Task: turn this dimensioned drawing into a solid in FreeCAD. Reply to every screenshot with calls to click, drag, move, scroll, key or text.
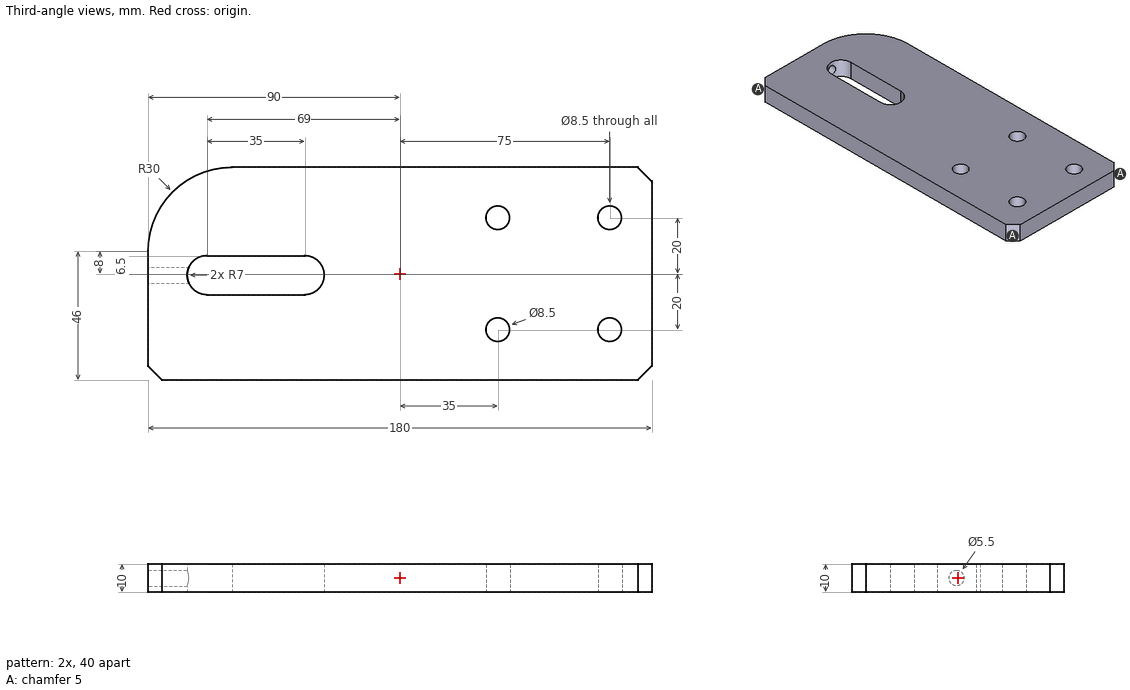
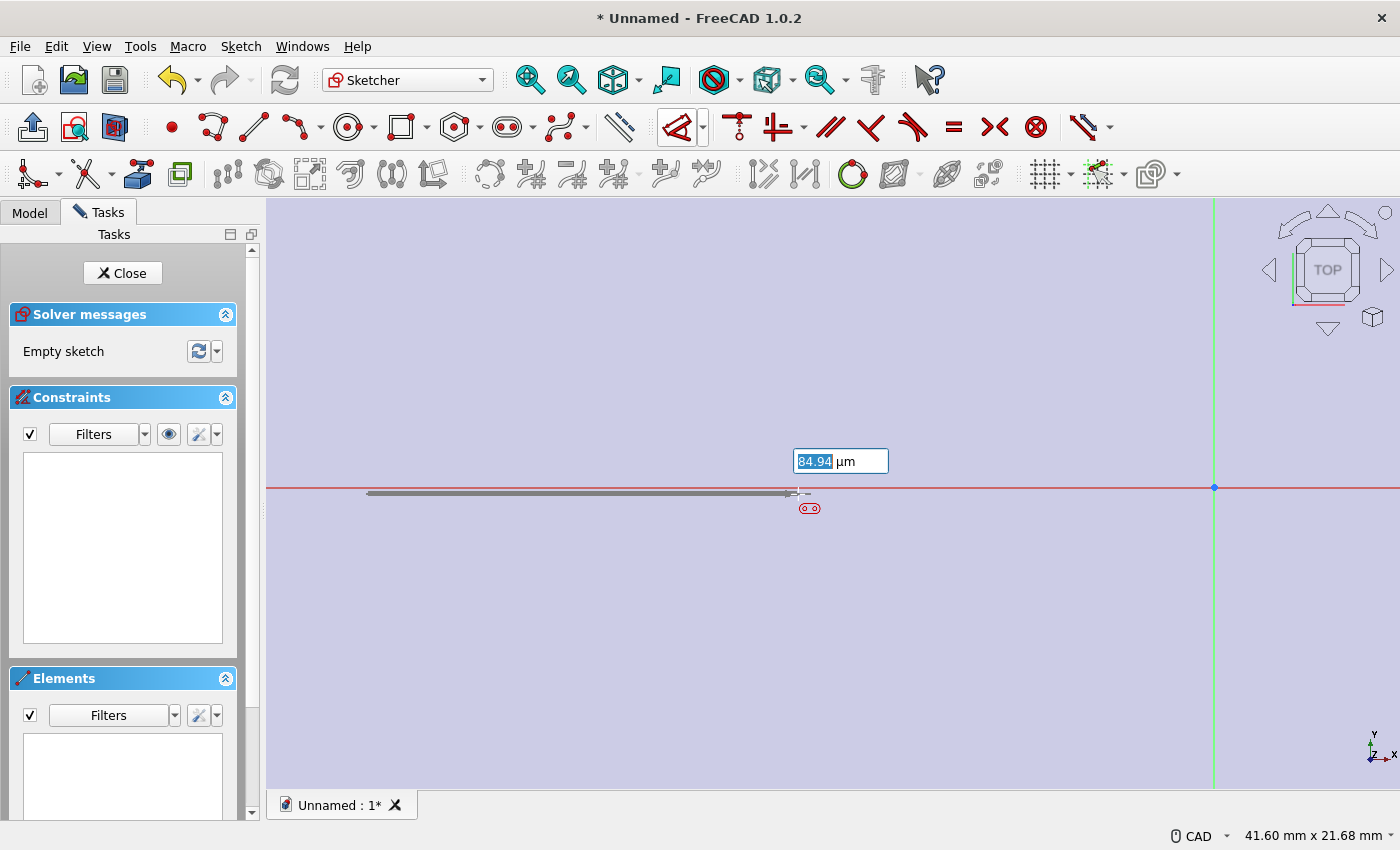
click(654, 436)
key(Escape)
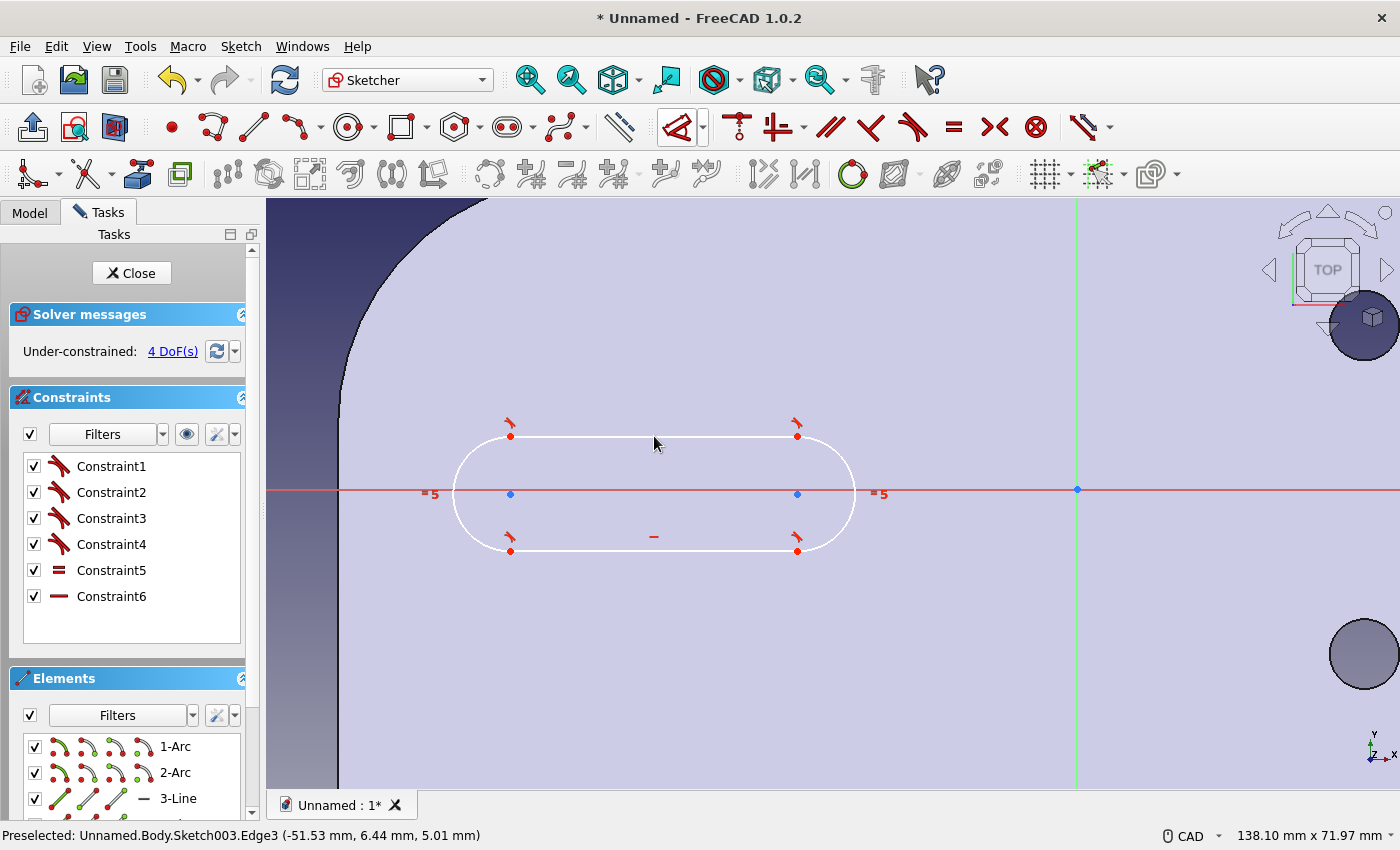
click(464, 461)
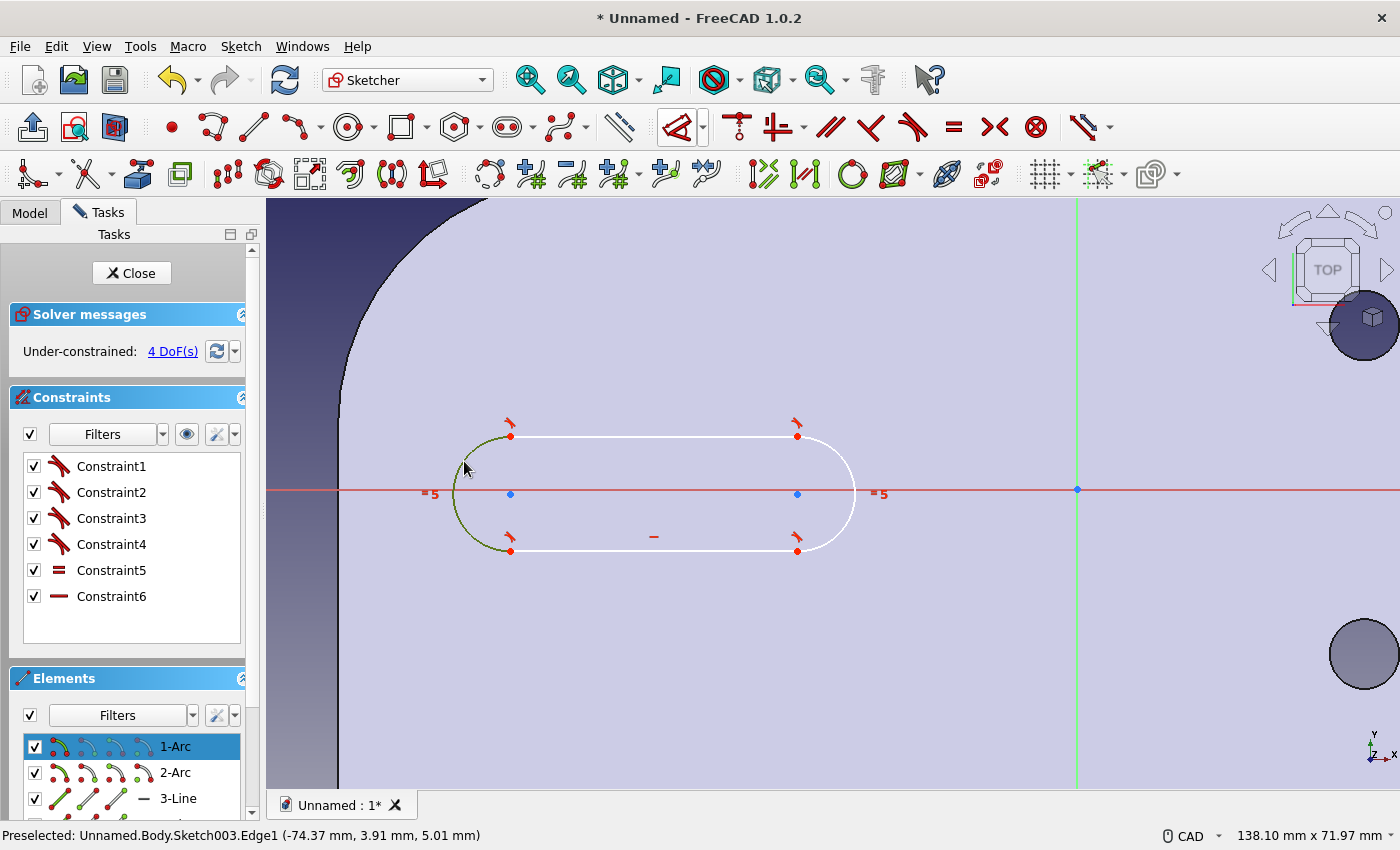
key(k)
key(r)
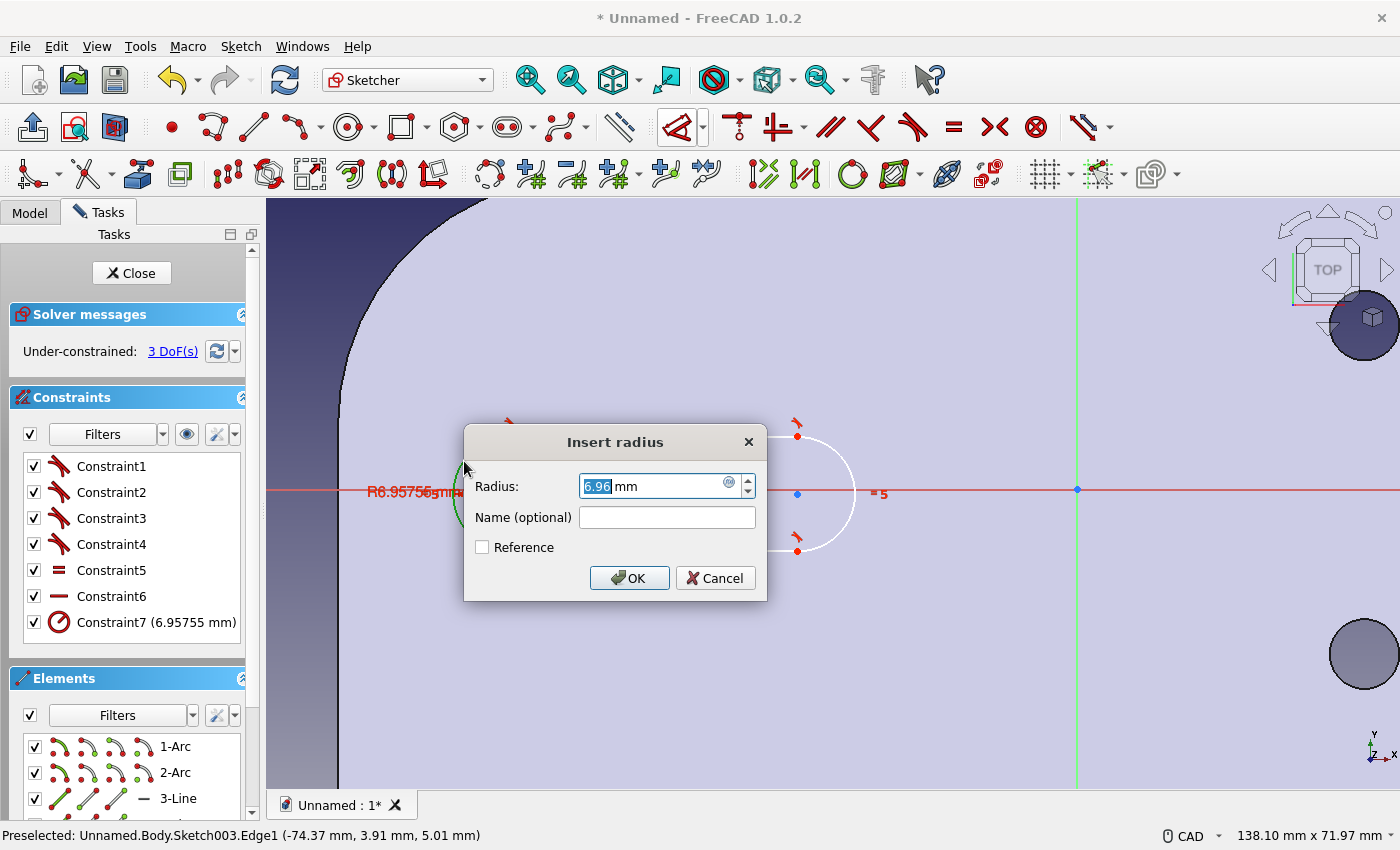
text(7)
key(Return)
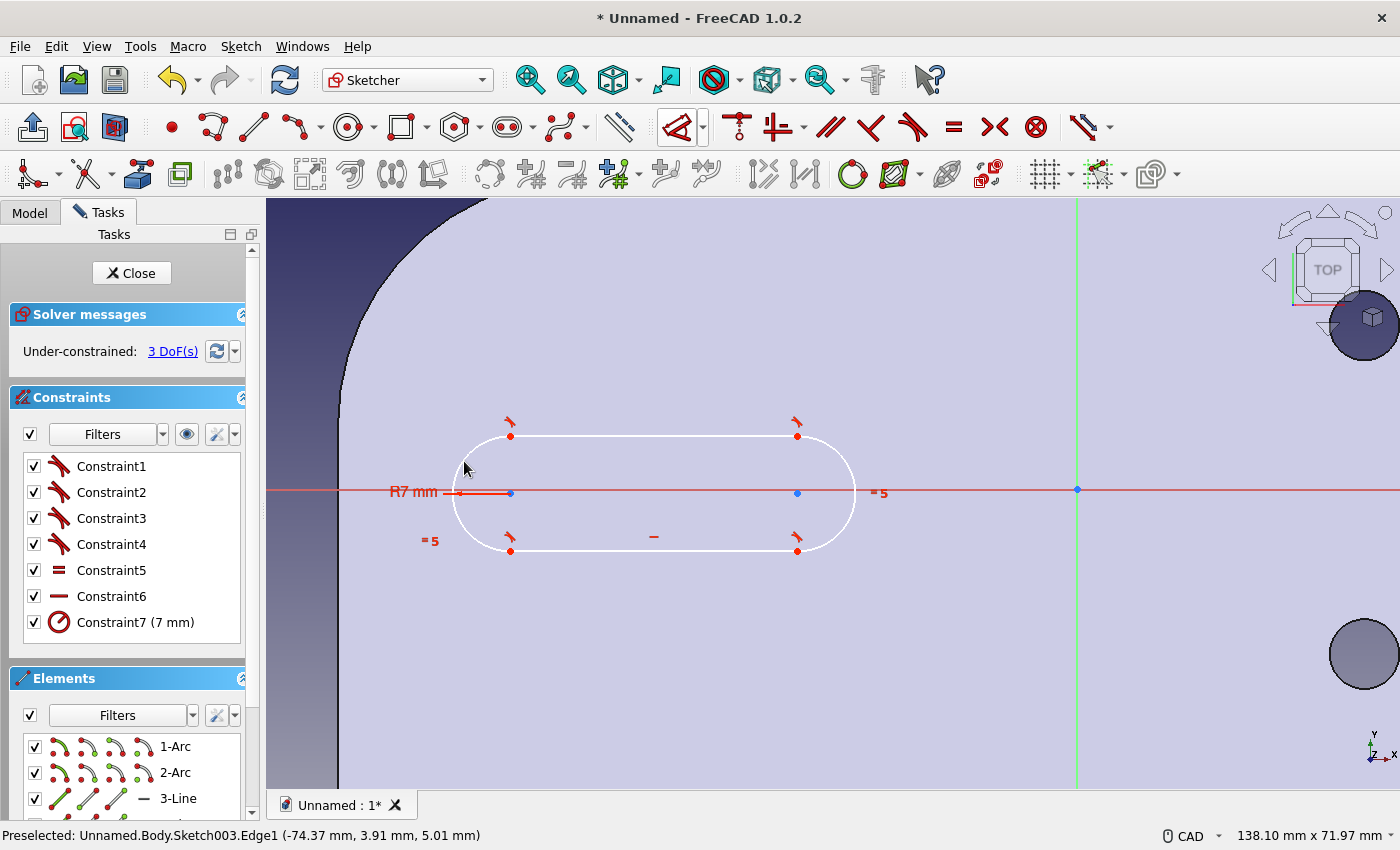
click(597, 436)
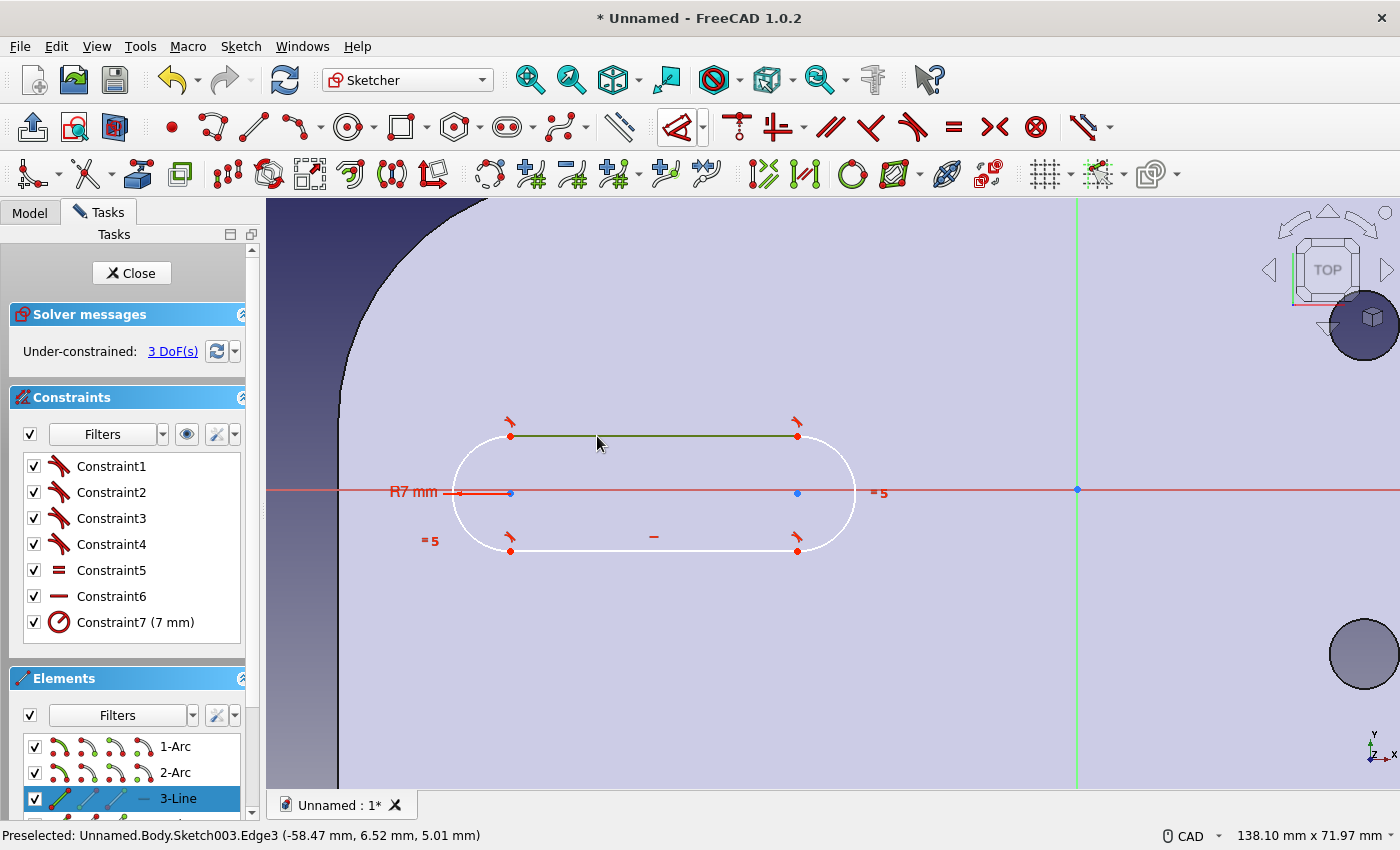
key(l)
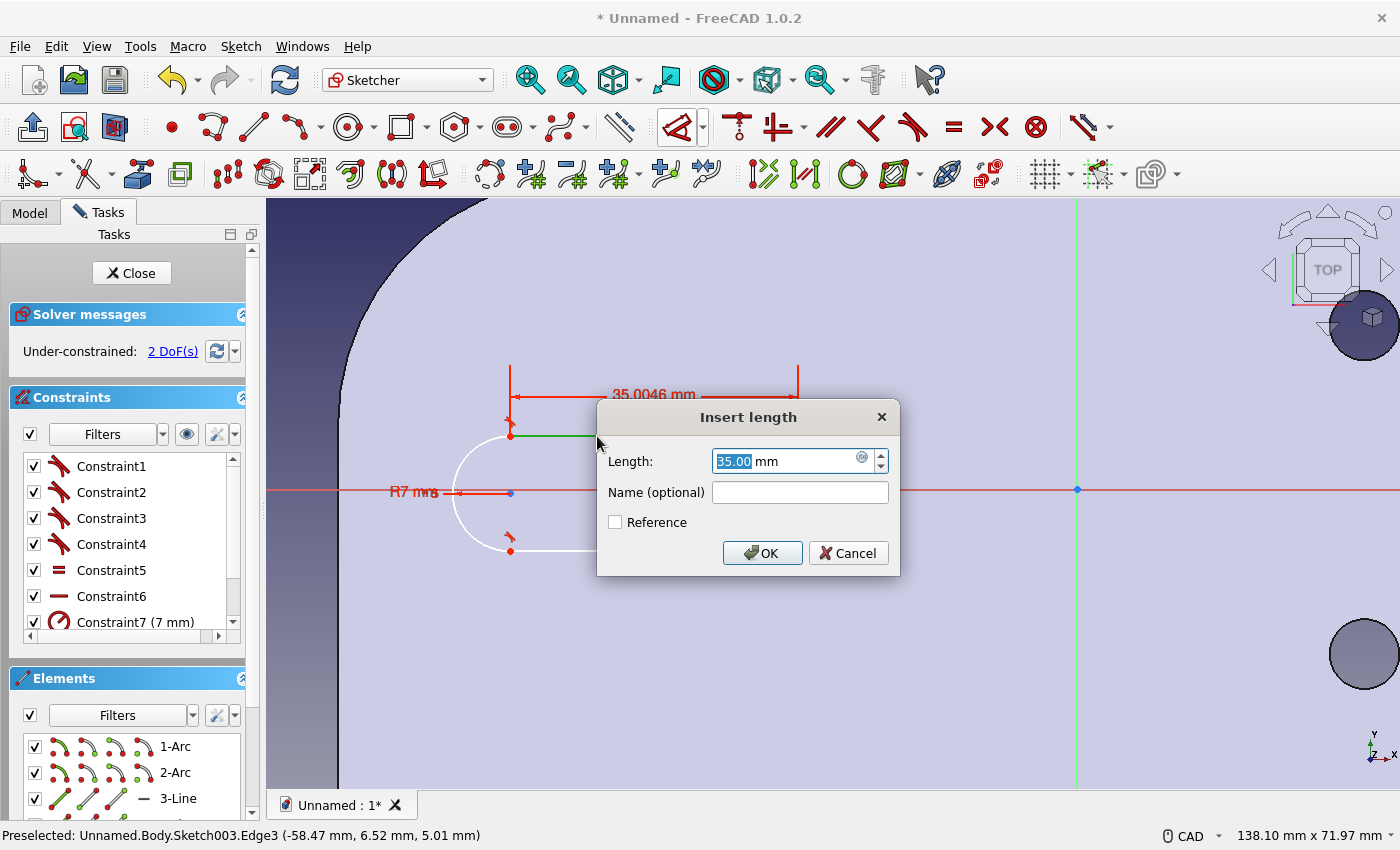
text(35)
key(Return)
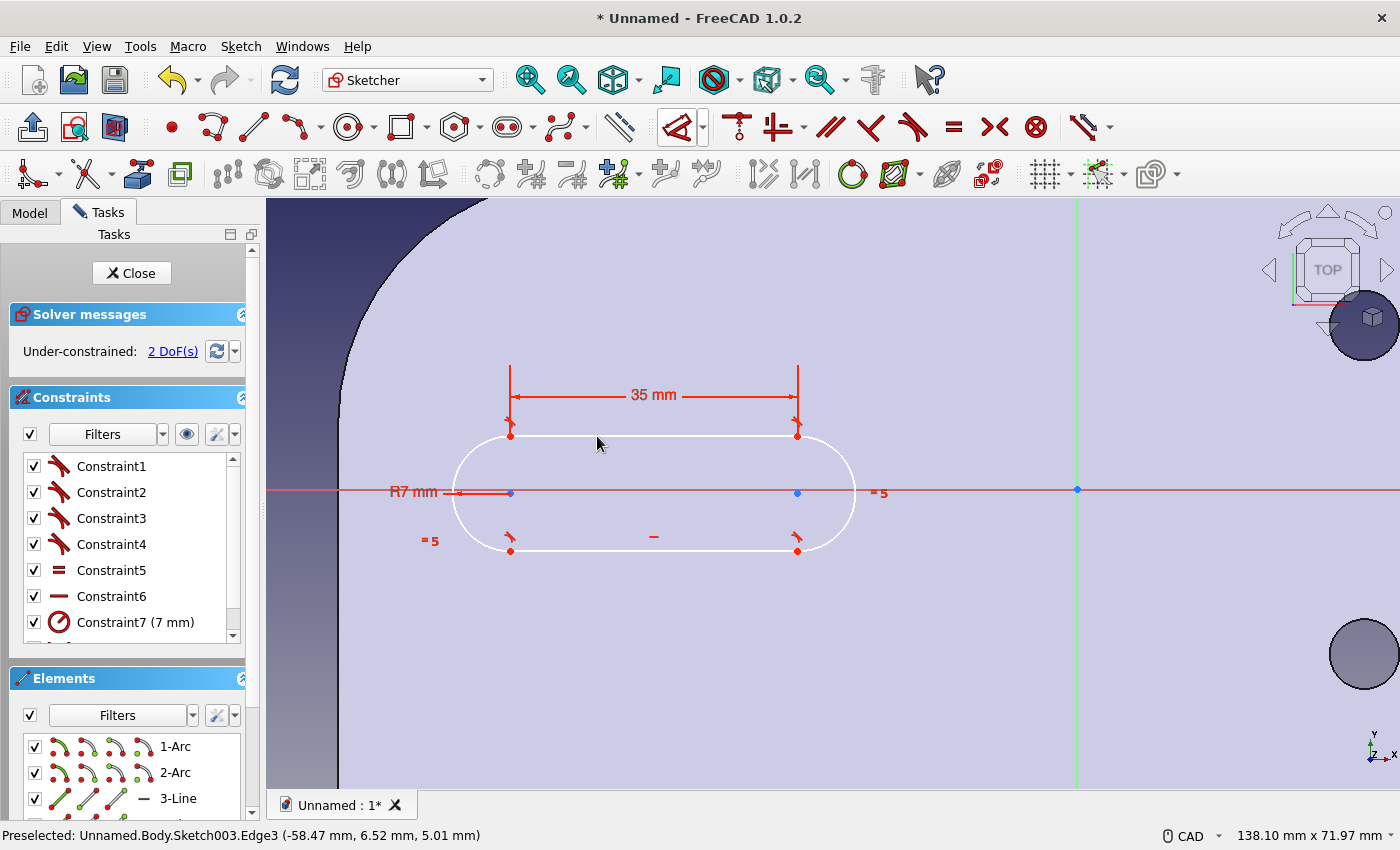
click(510, 436)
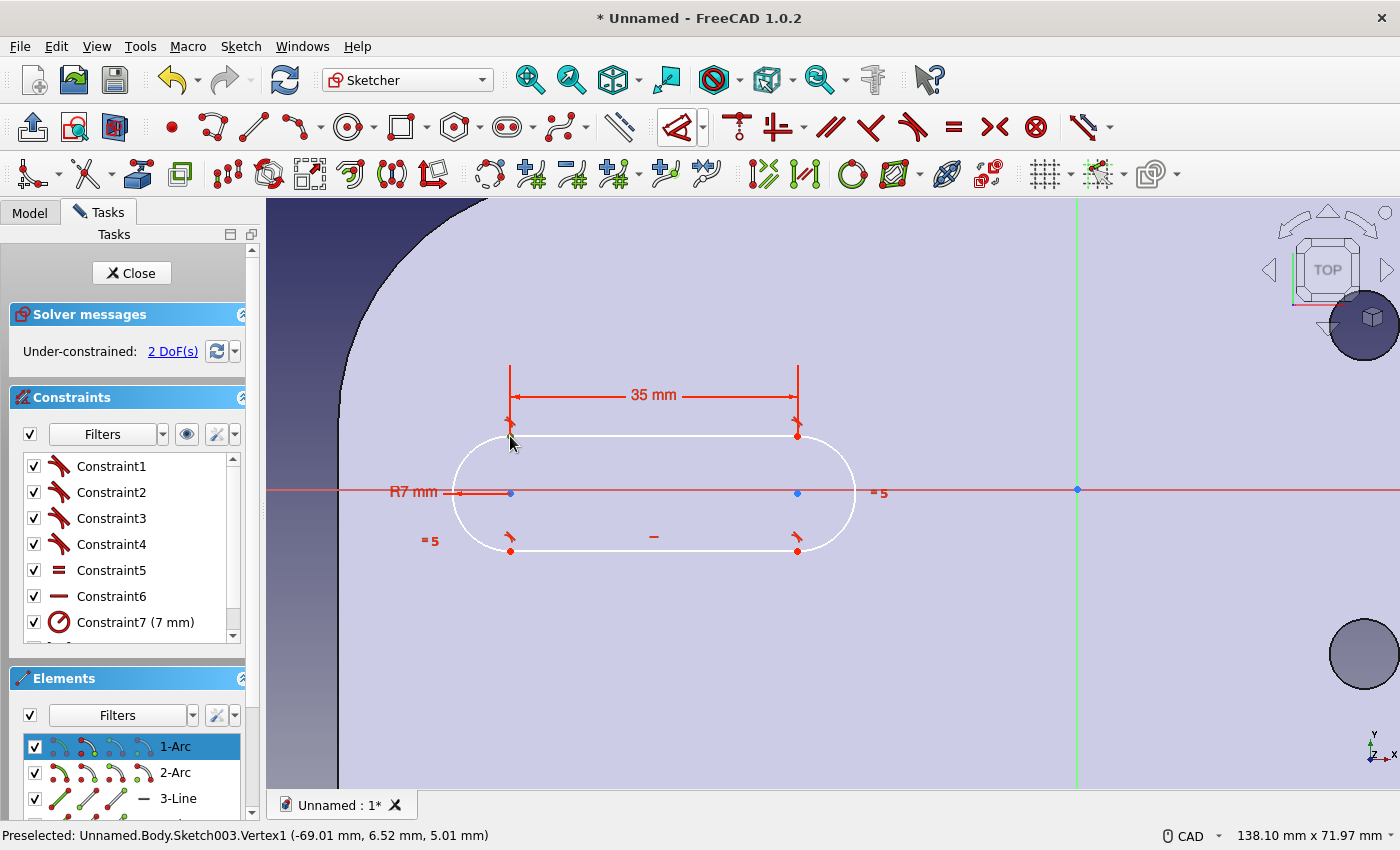
click(702, 128)